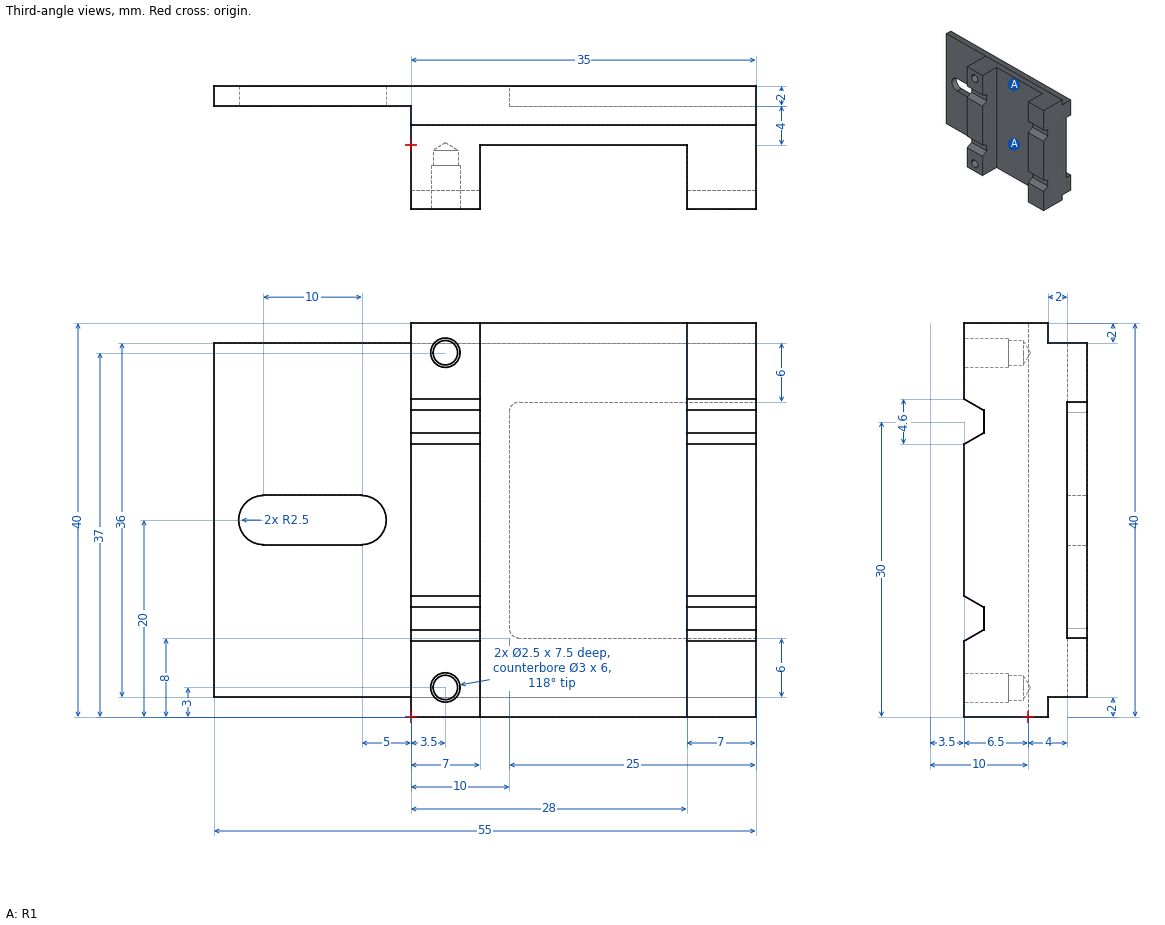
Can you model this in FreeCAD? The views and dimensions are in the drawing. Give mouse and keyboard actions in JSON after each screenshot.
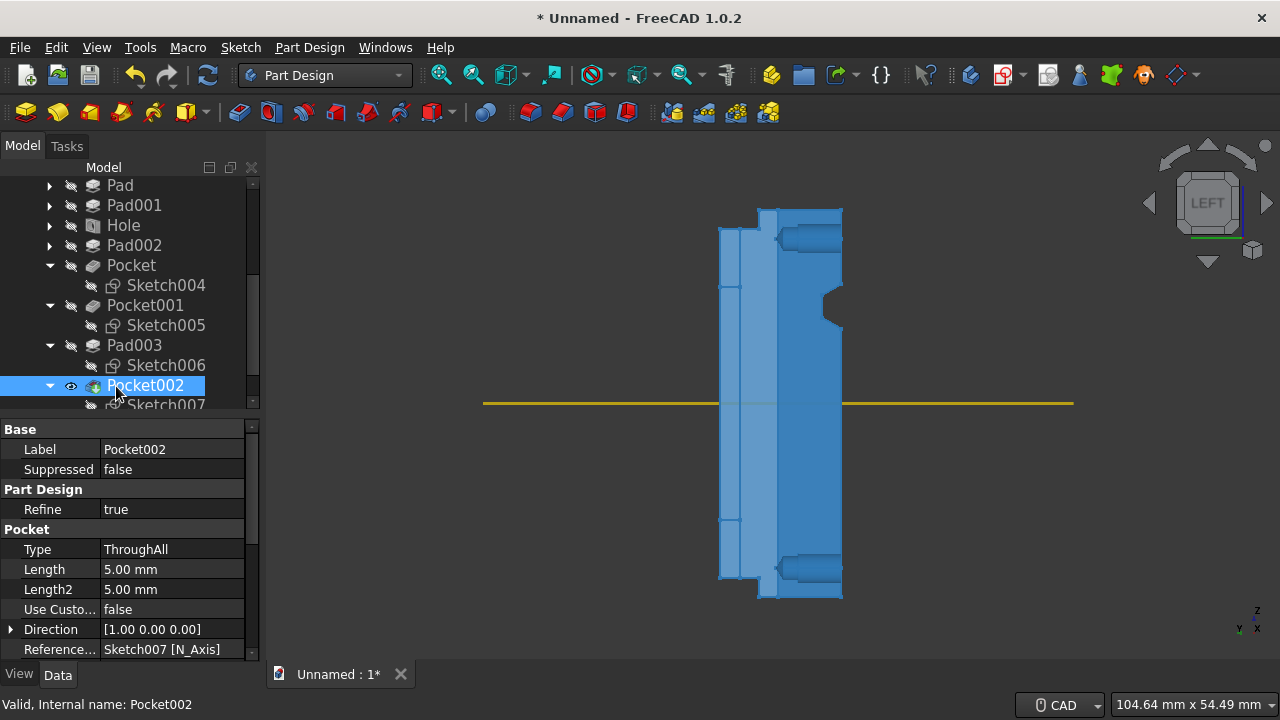
{"action": "left_click", "coordinate": [672, 112]}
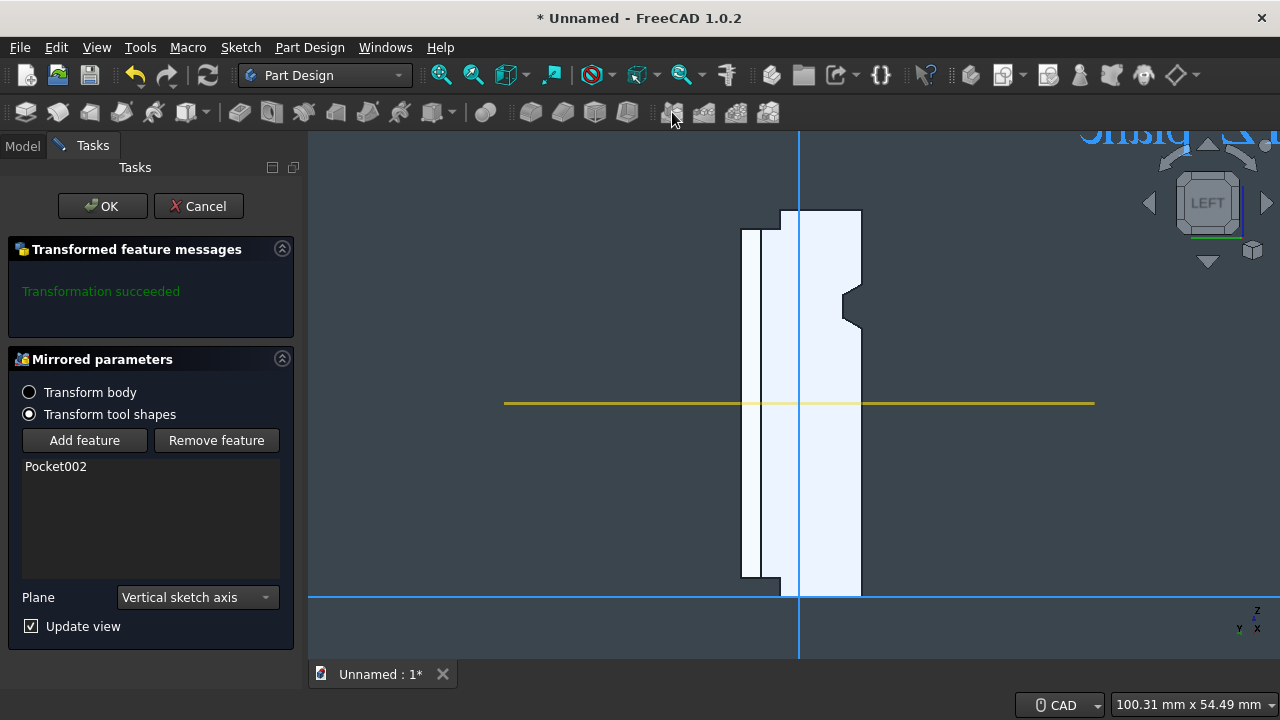
{"action": "left_click", "coordinate": [198, 598]}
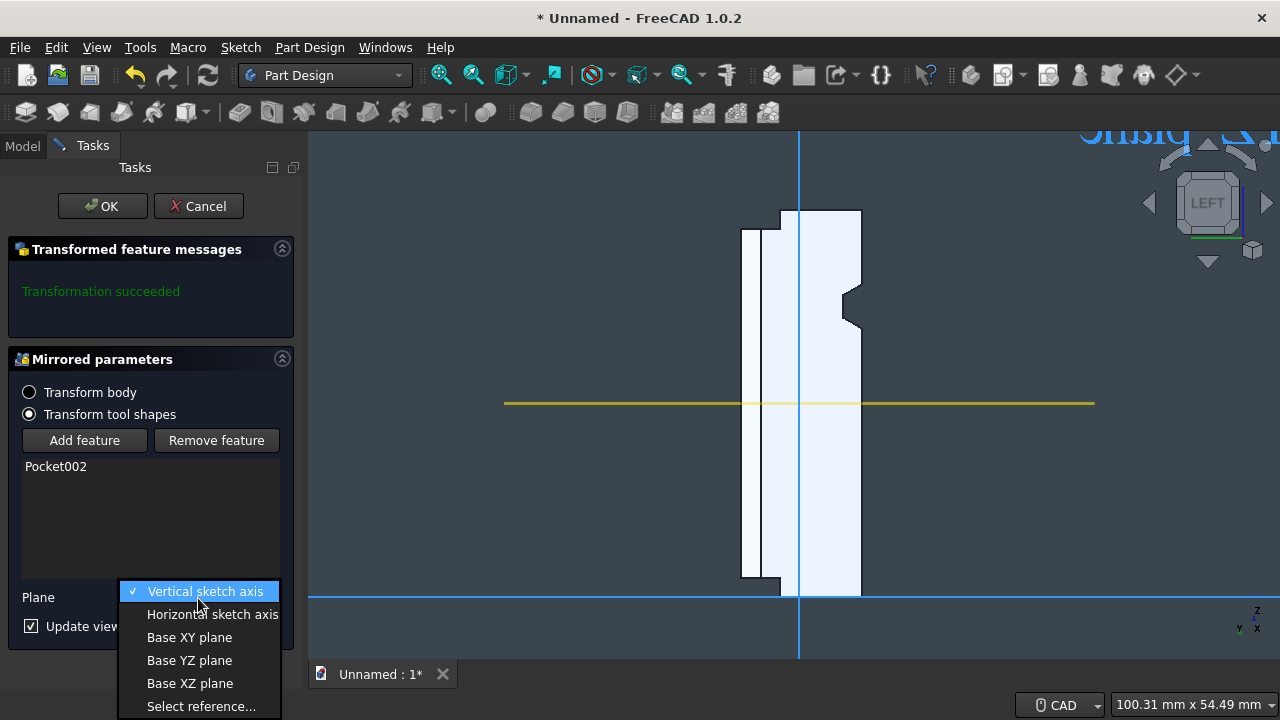
{"action": "left_click", "coordinate": [198, 706]}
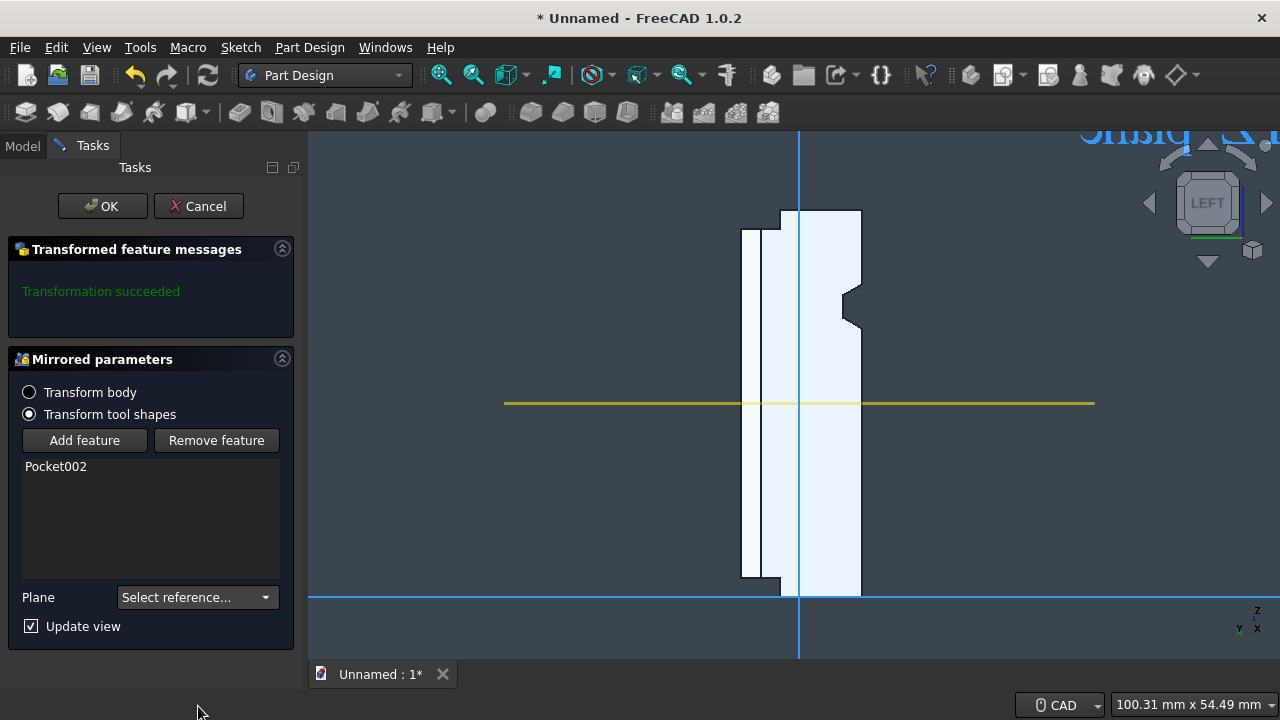
{"action": "left_click", "coordinate": [23, 145]}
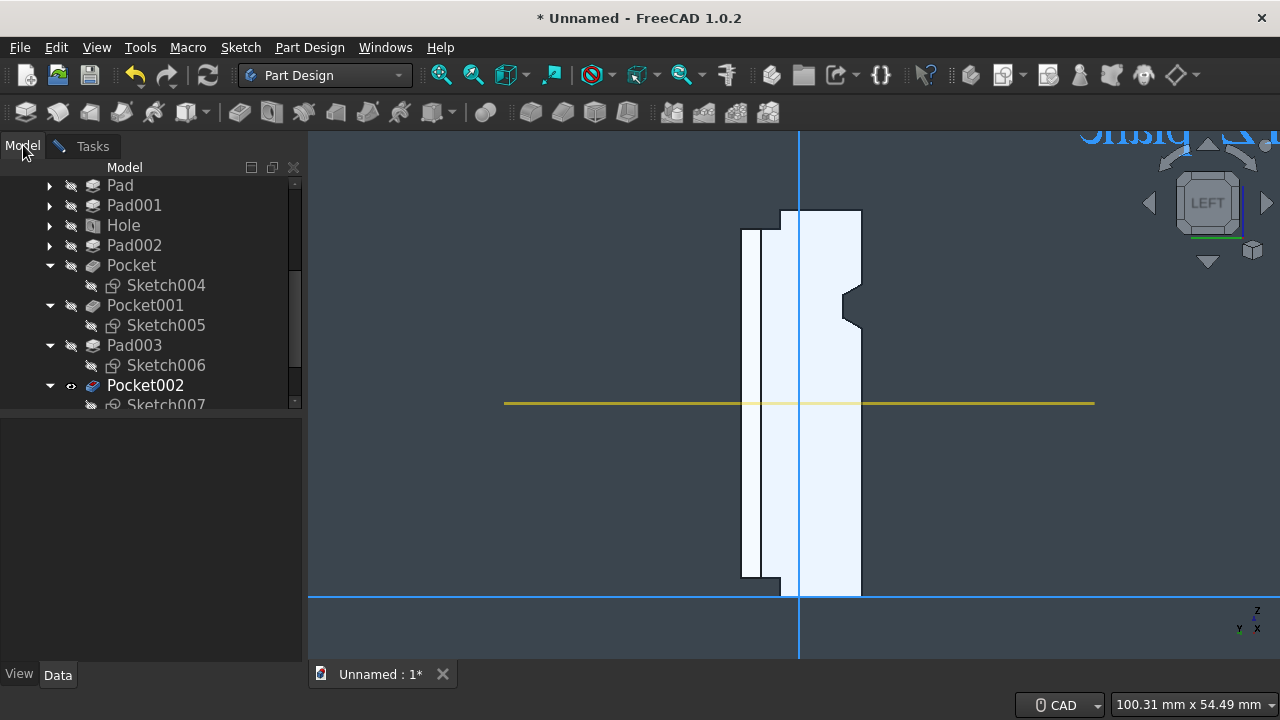
{"action": "scroll", "coordinate": [140, 301], "scroll_direction": "down", "scroll_amount": 3}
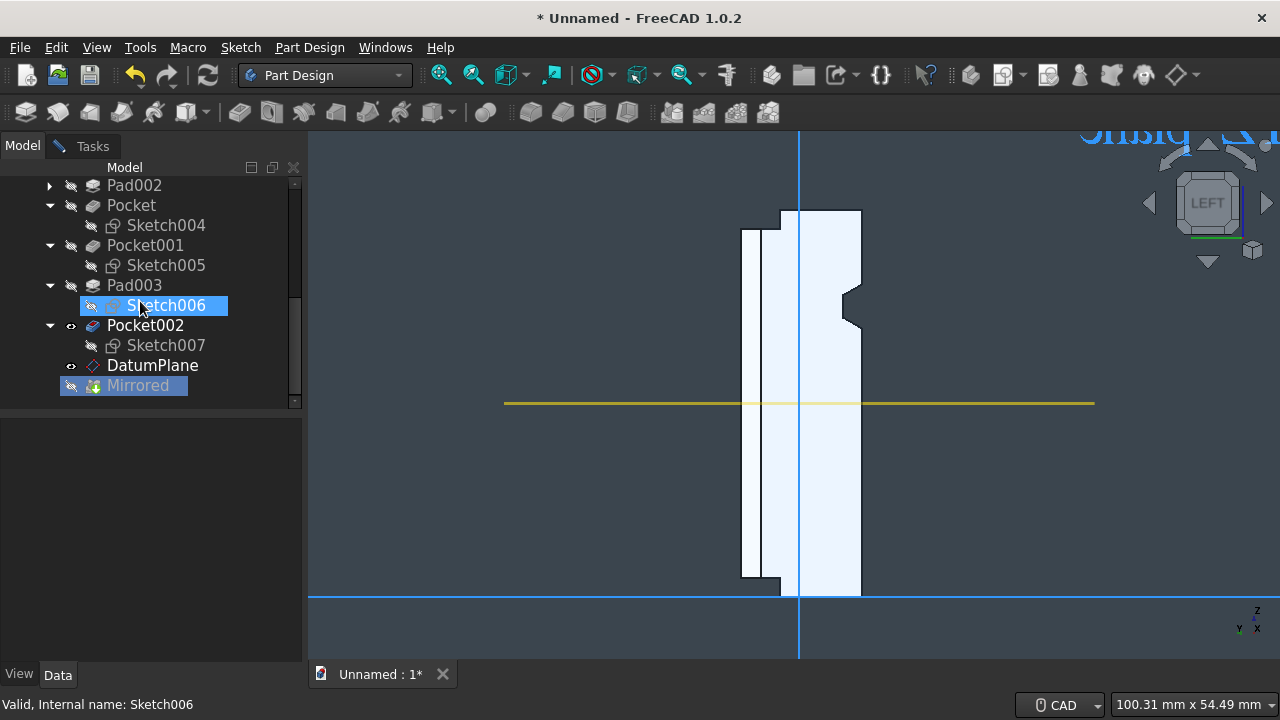
{"action": "left_click", "coordinate": [116, 366]}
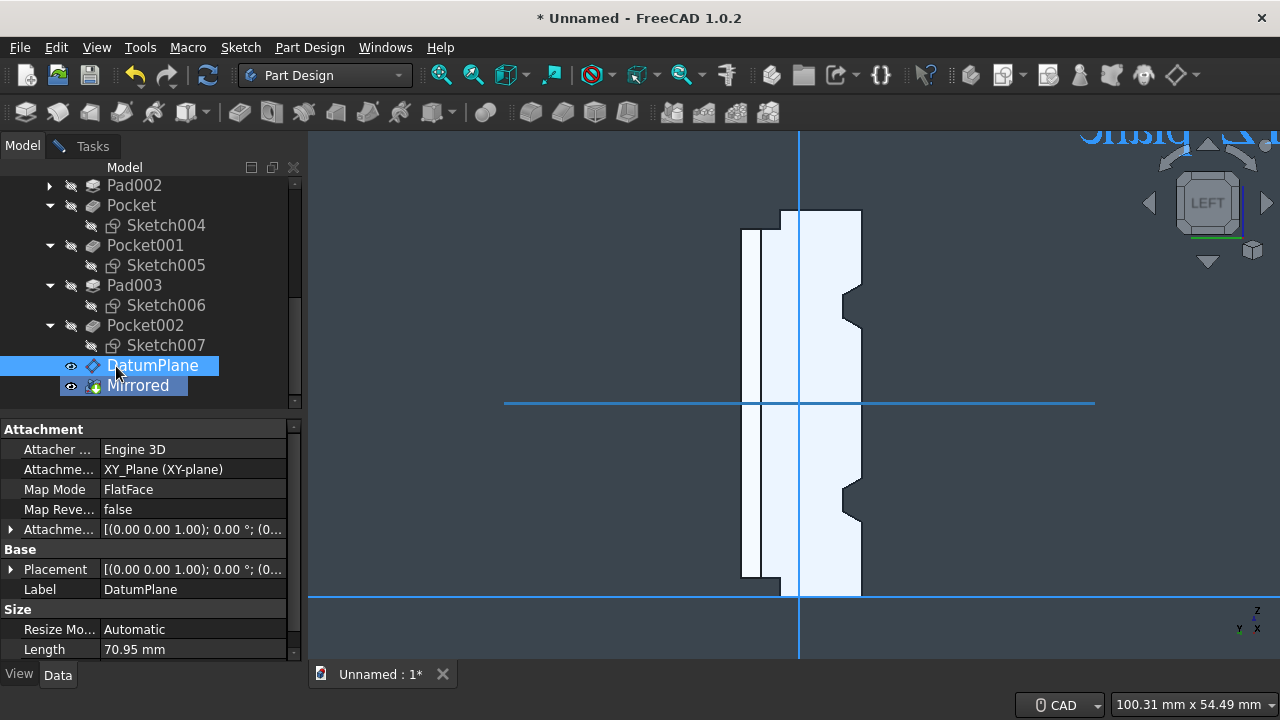
{"action": "left_click", "coordinate": [84, 145]}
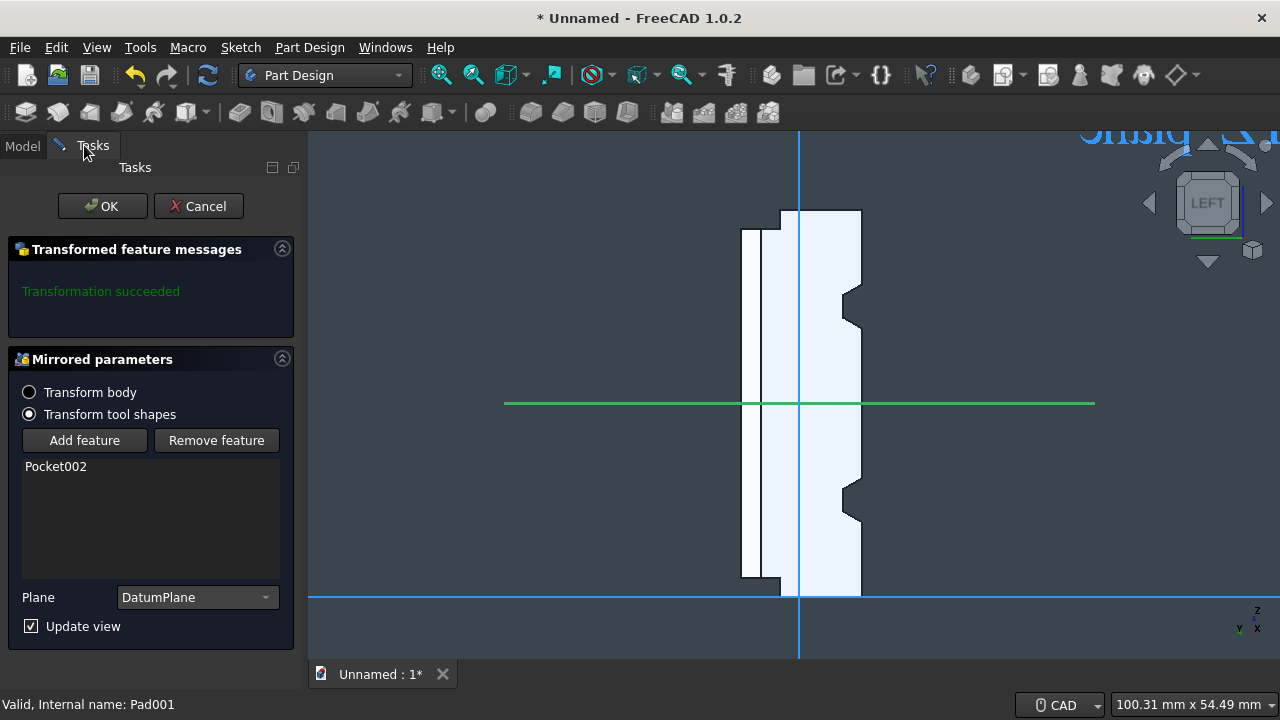
{"action": "left_click", "coordinate": [103, 206]}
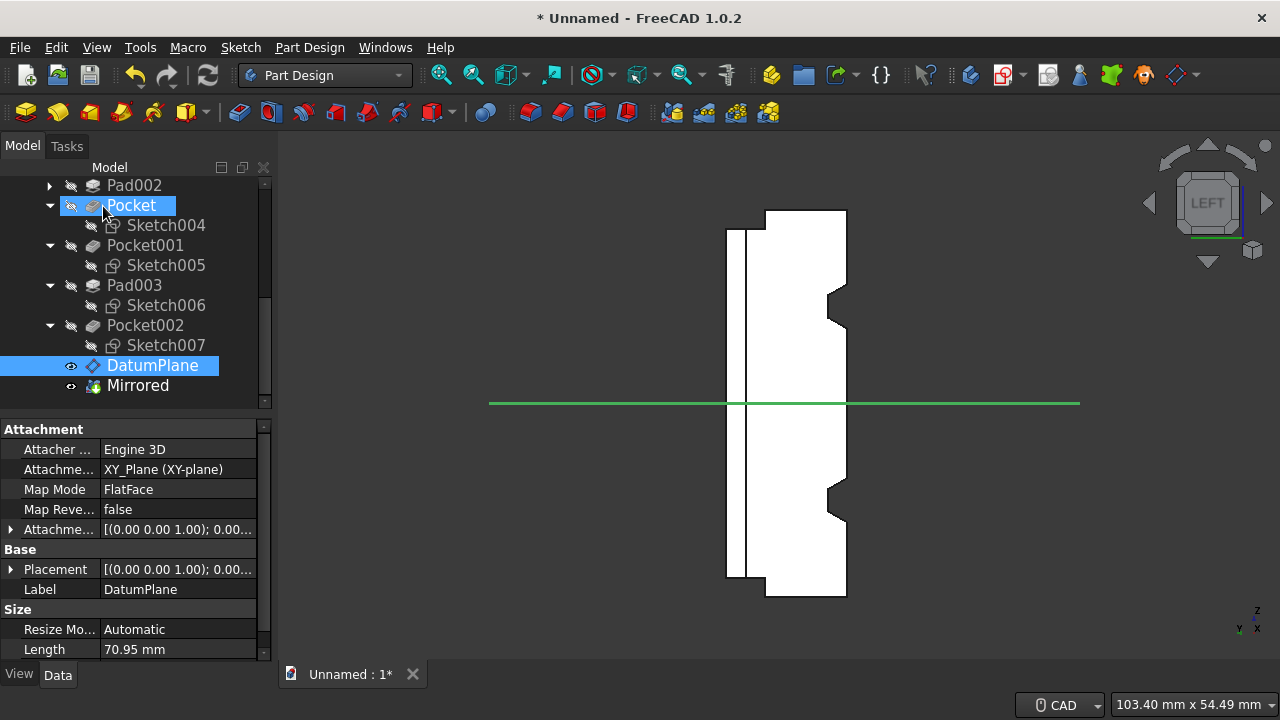
{"action": "left_click", "coordinate": [116, 366]}
{"action": "key", "text": "space"}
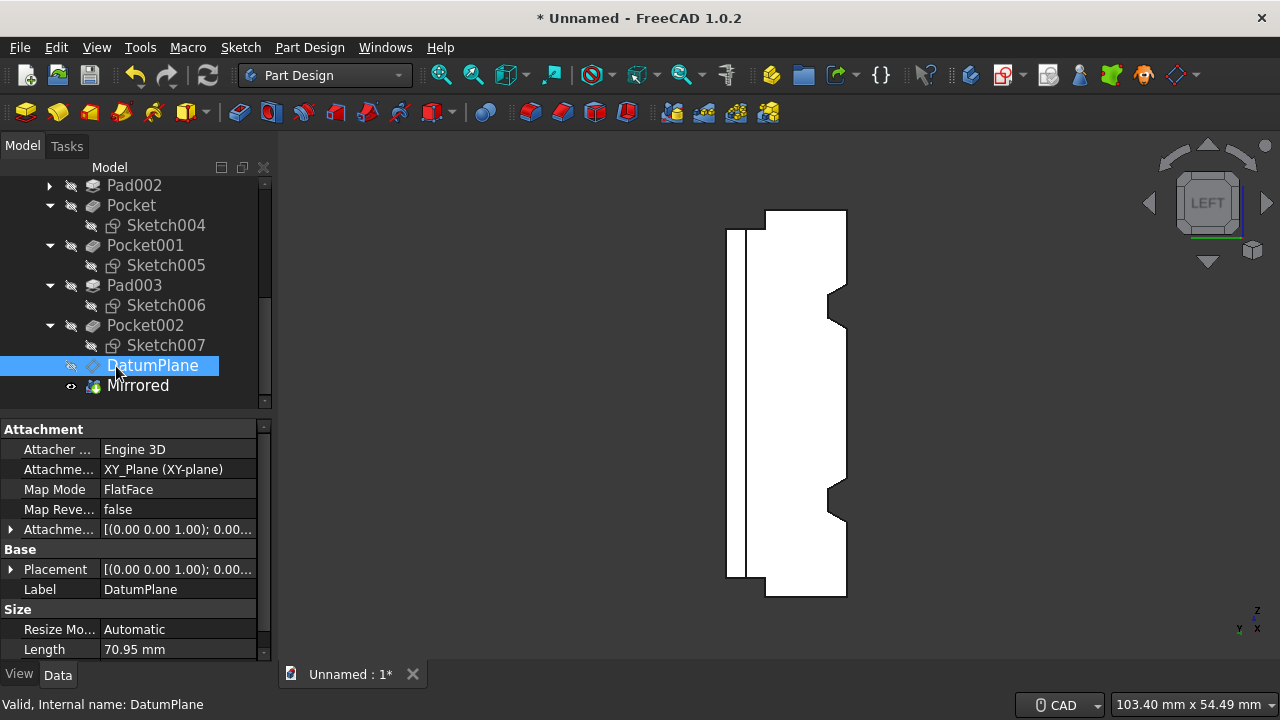
{"action": "scroll", "coordinate": [736, 286], "scroll_direction": "up", "scroll_amount": 4}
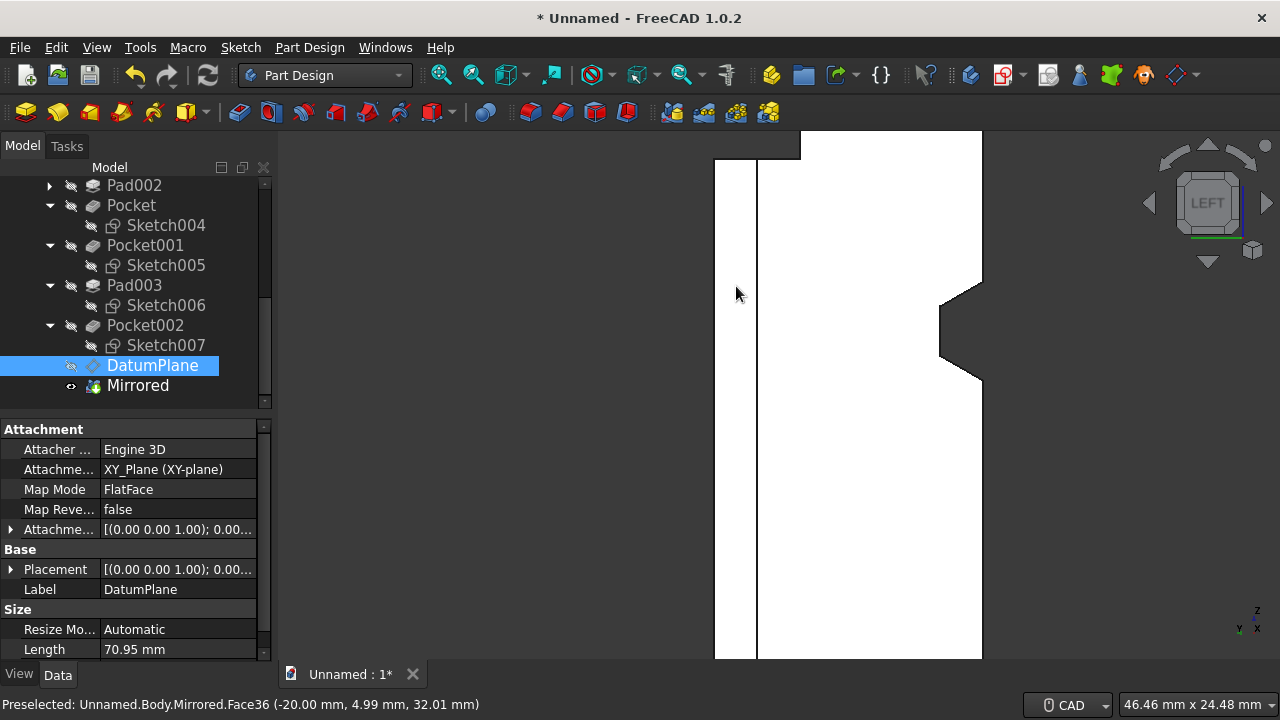
{"action": "left_click", "coordinate": [442, 76]}